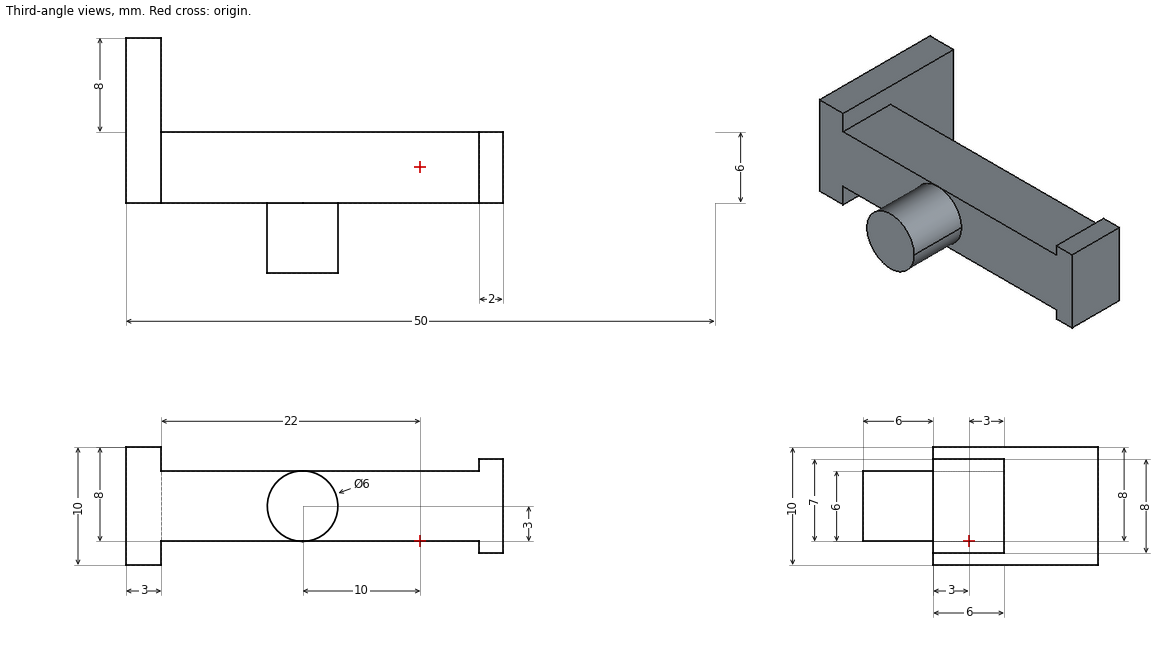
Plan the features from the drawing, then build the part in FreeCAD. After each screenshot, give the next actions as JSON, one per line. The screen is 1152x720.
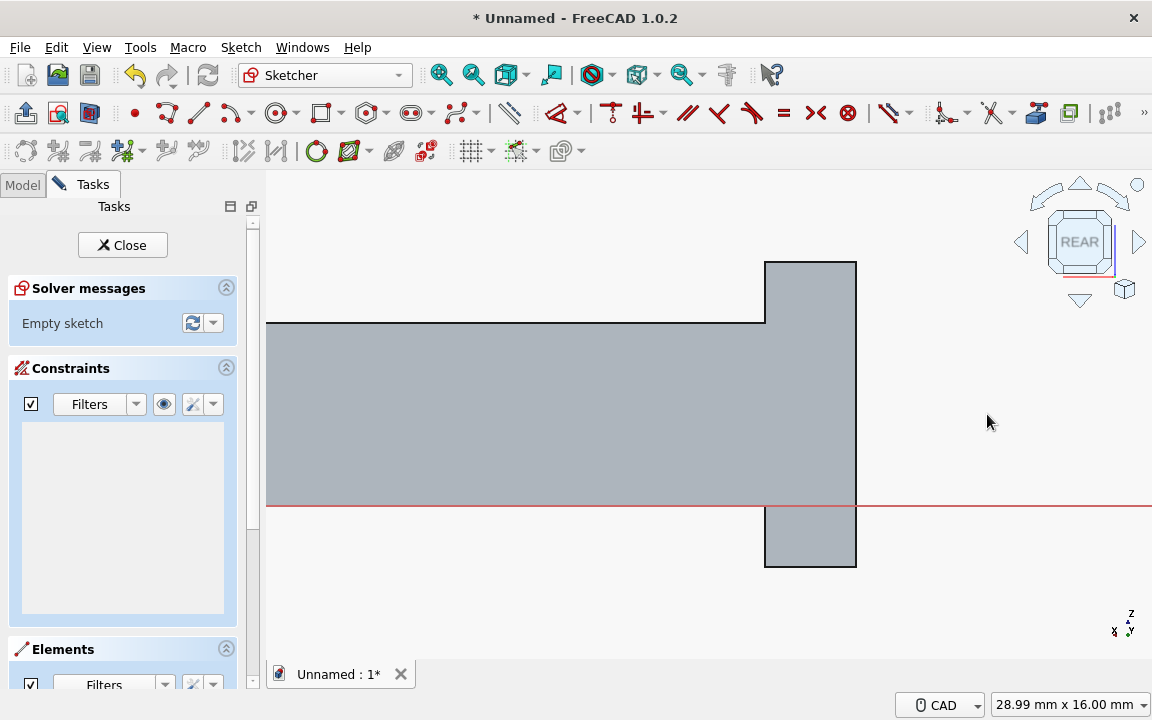
{"action": "left_click", "coordinate": [322, 114]}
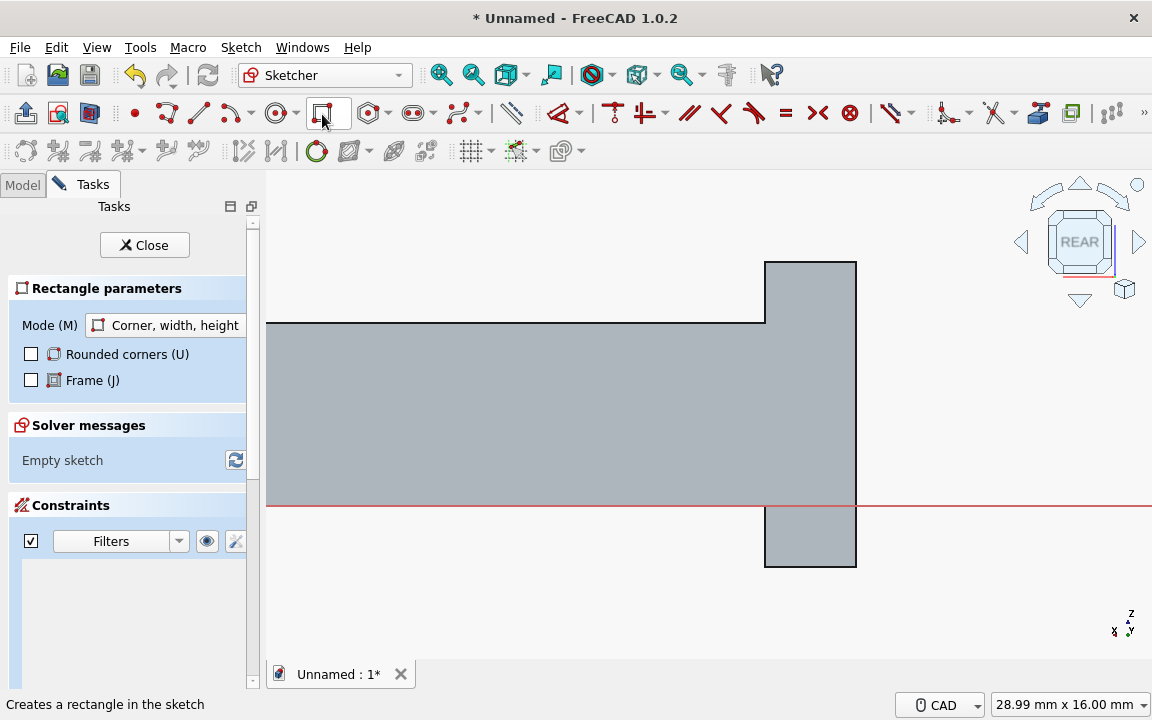
{"action": "left_click", "coordinate": [765, 262]}
{"action": "mouse_move", "coordinate": [856, 567]}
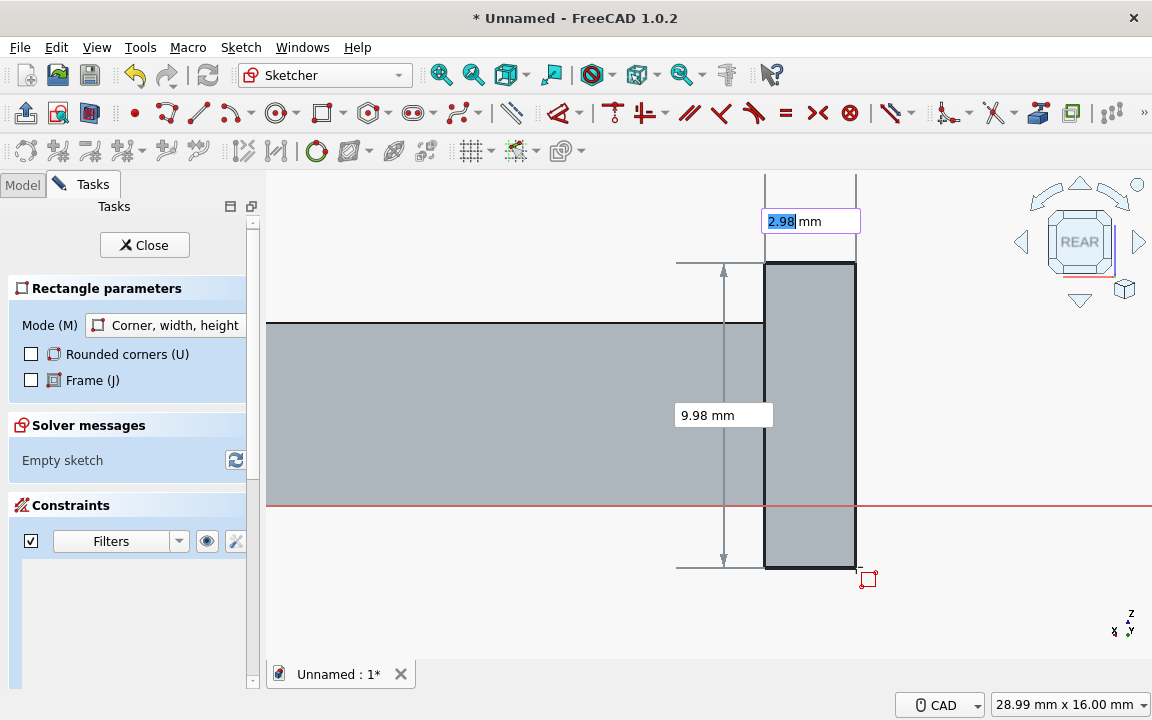
{"action": "type", "text": "3"}
{"action": "key", "text": "Tab"}
{"action": "type", "text": "10"}
{"action": "key", "text": "Return"}
{"action": "key", "text": "Escape"}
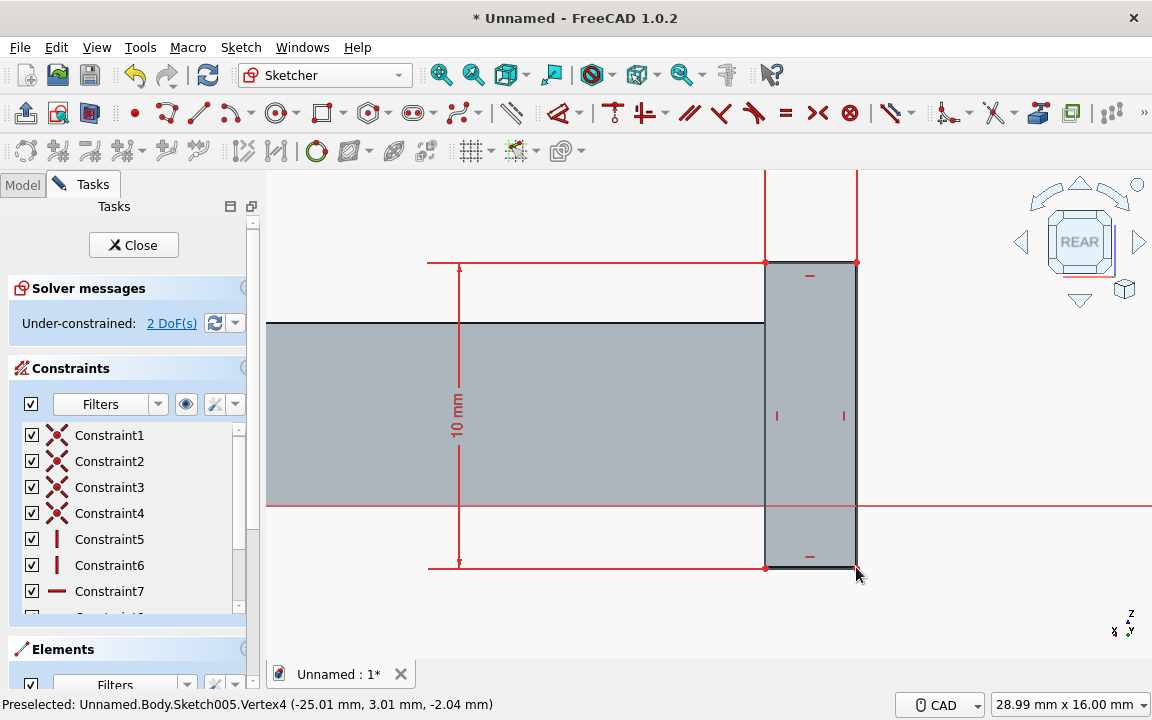
{"action": "left_click", "coordinate": [558, 114]}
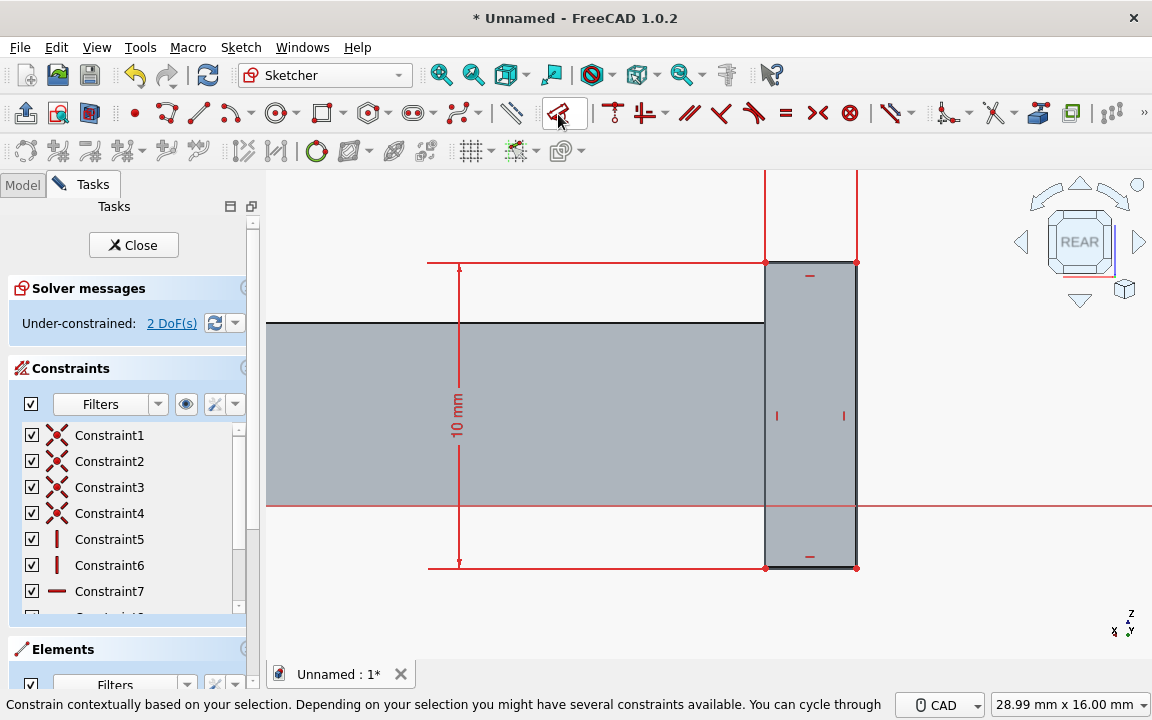
{"action": "left_click", "coordinate": [765, 263]}
{"action": "left_click", "coordinate": [799, 385]}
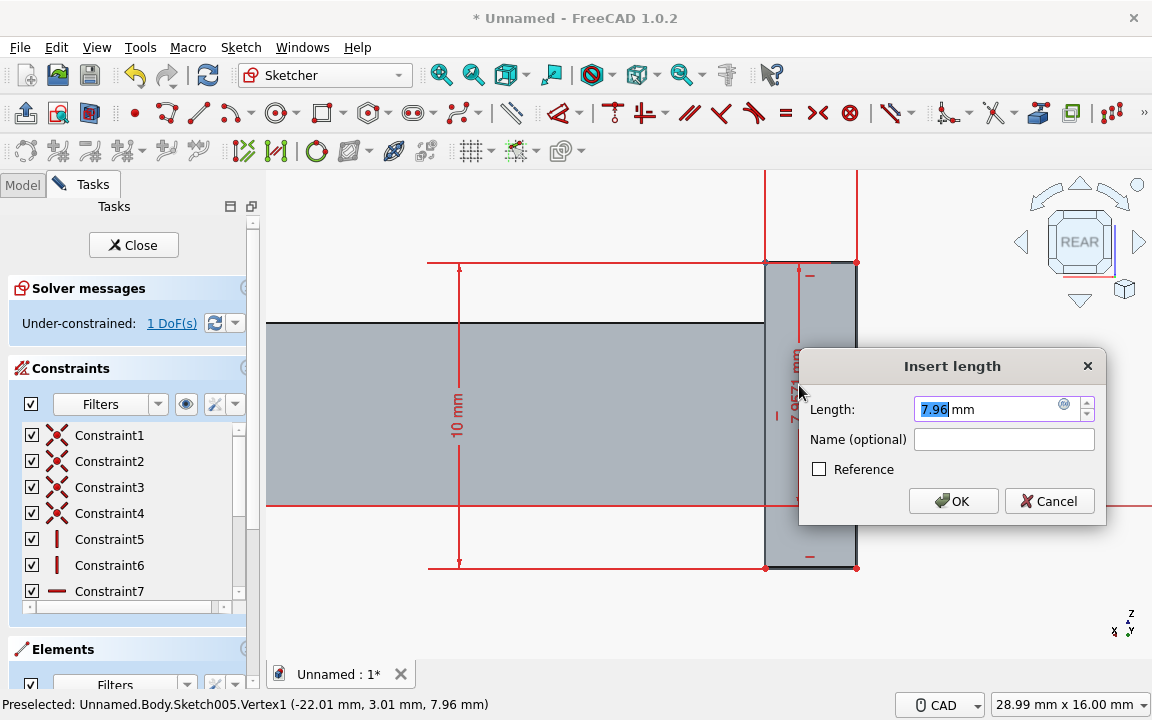
{"action": "type", "text": "8"}
{"action": "key", "text": "Return"}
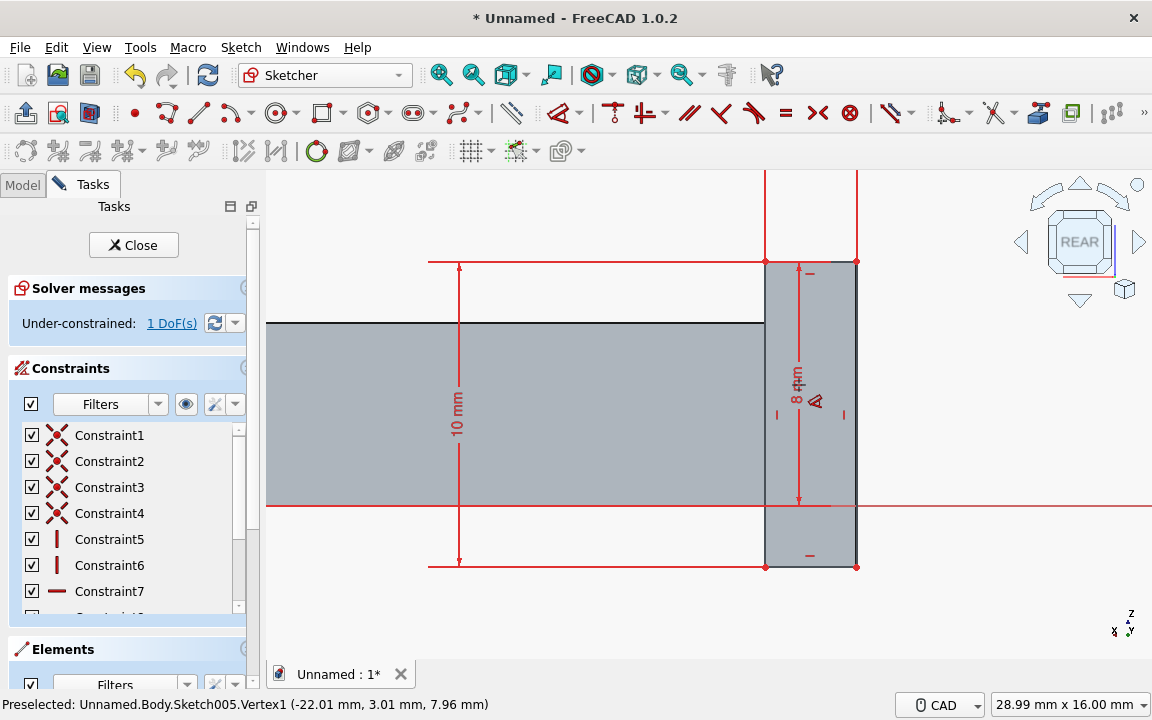
{"action": "left_click", "coordinate": [765, 262]}
{"action": "left_click", "coordinate": [530, 228]}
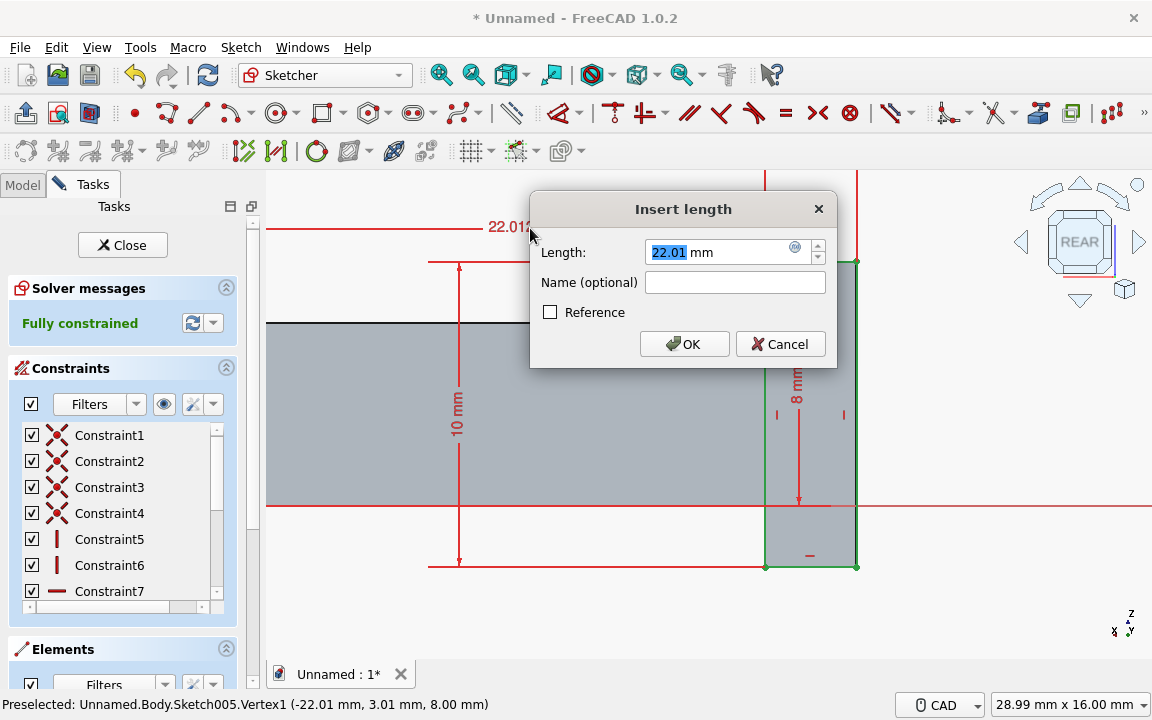
{"action": "type", "text": "22"}
{"action": "key", "text": "Return"}
{"action": "key", "text": "Escape"}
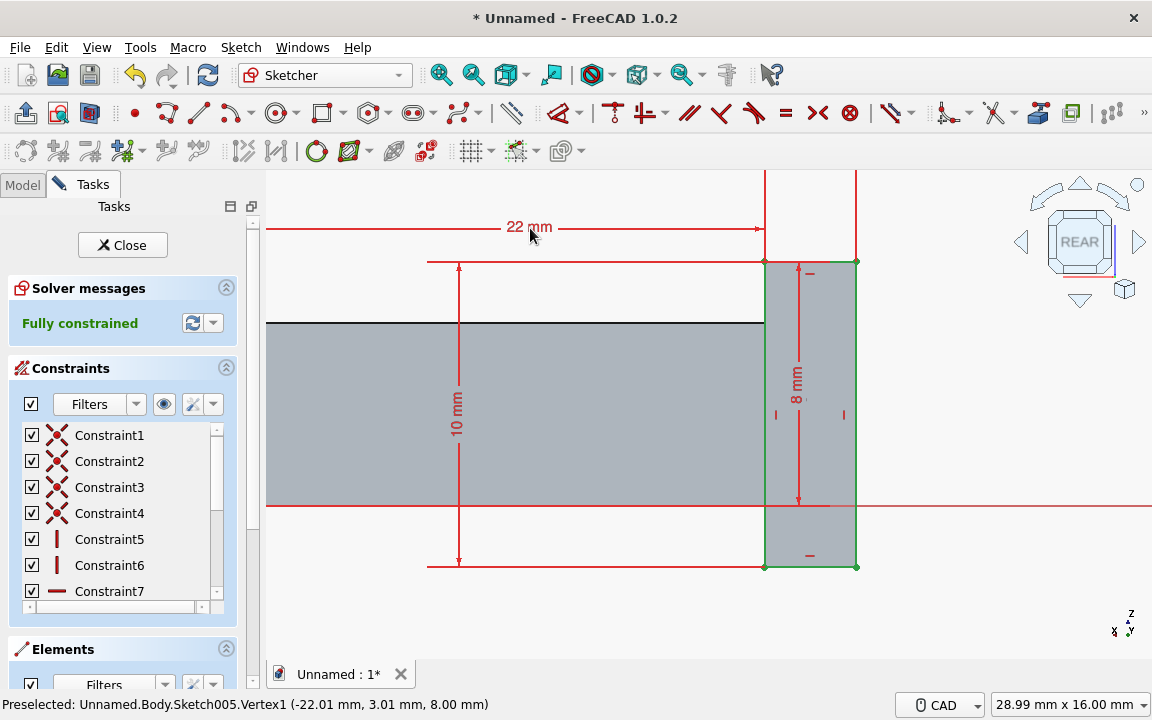
{"action": "left_click", "coordinate": [123, 245]}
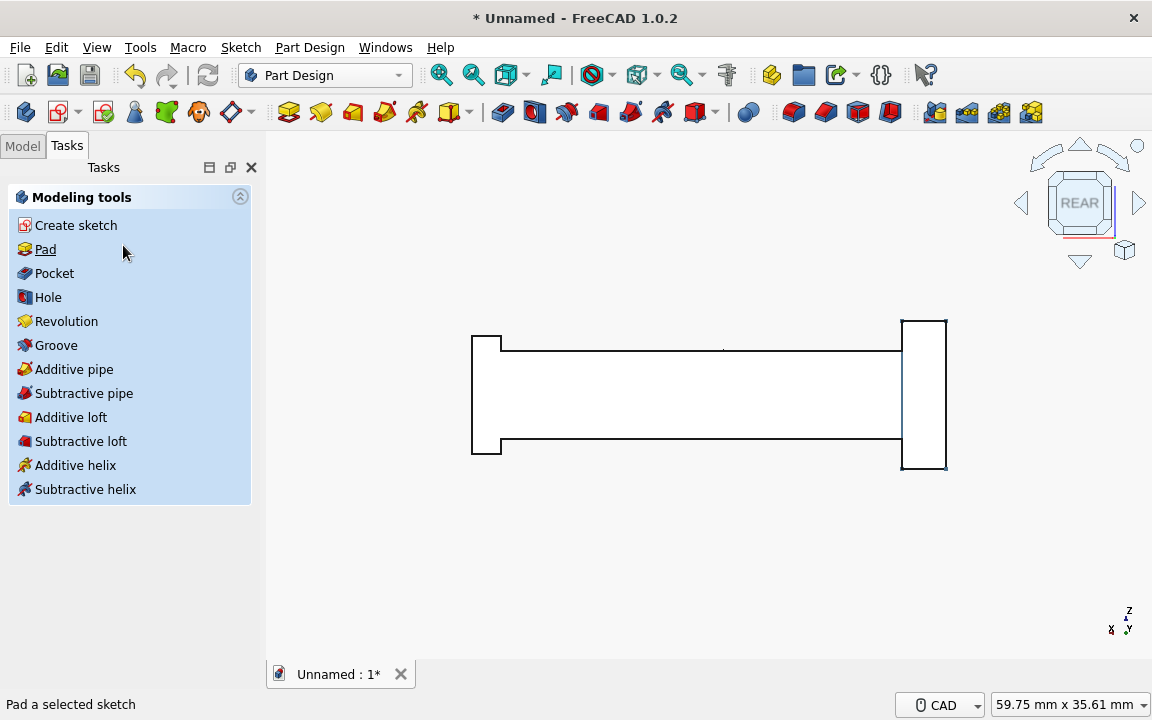
{"action": "left_click", "coordinate": [290, 112]}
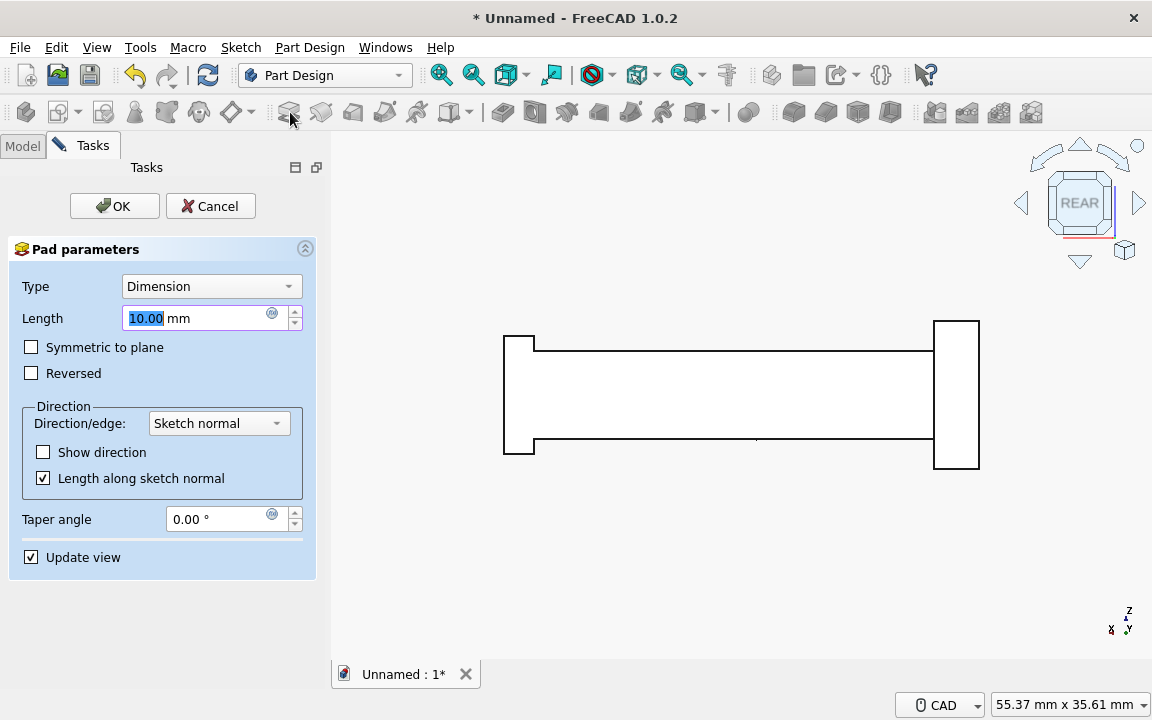
{"action": "type", "text": "8"}
{"action": "key", "text": "Tab"}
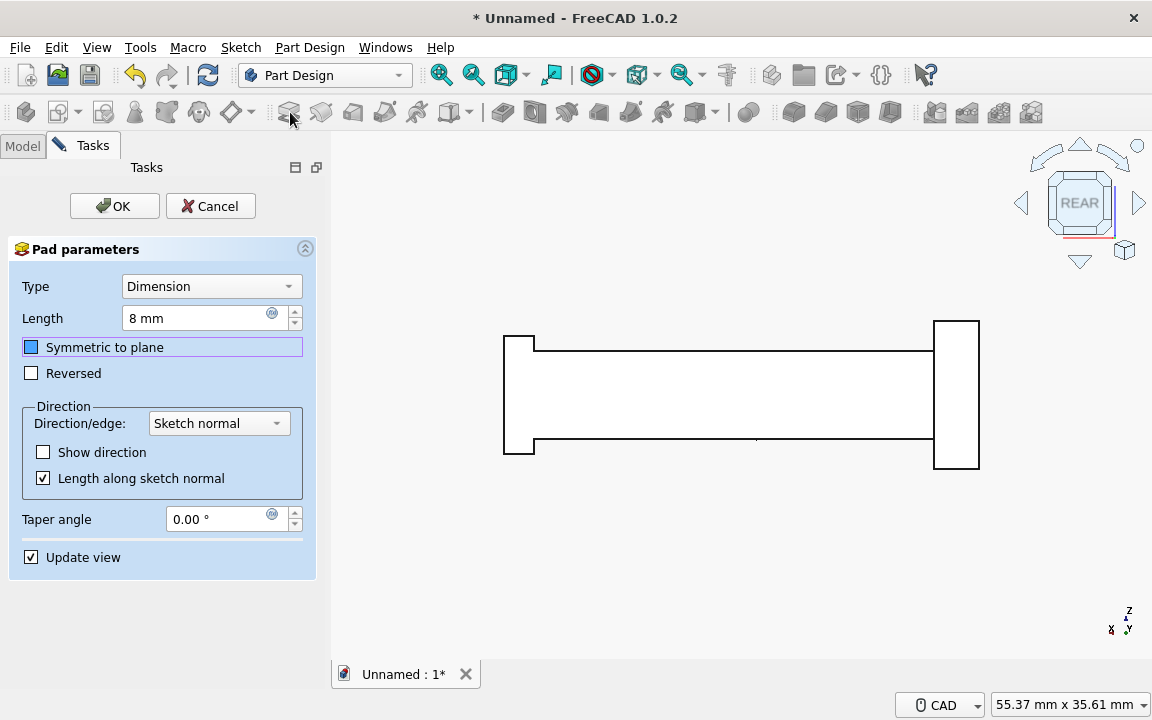
{"action": "left_click", "coordinate": [115, 206]}